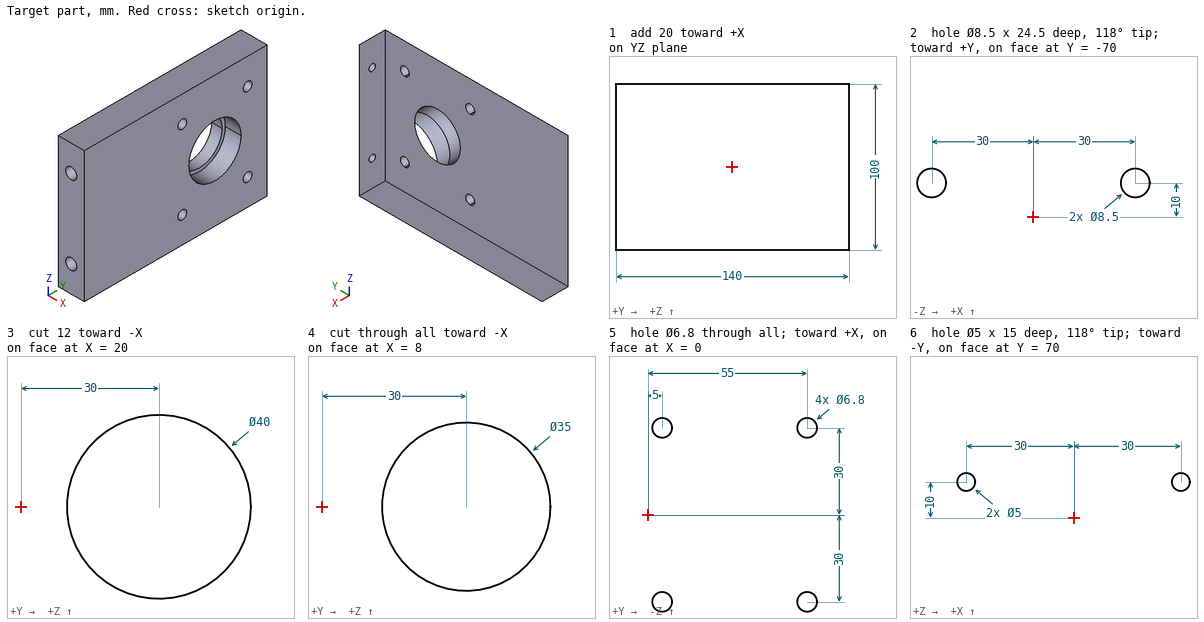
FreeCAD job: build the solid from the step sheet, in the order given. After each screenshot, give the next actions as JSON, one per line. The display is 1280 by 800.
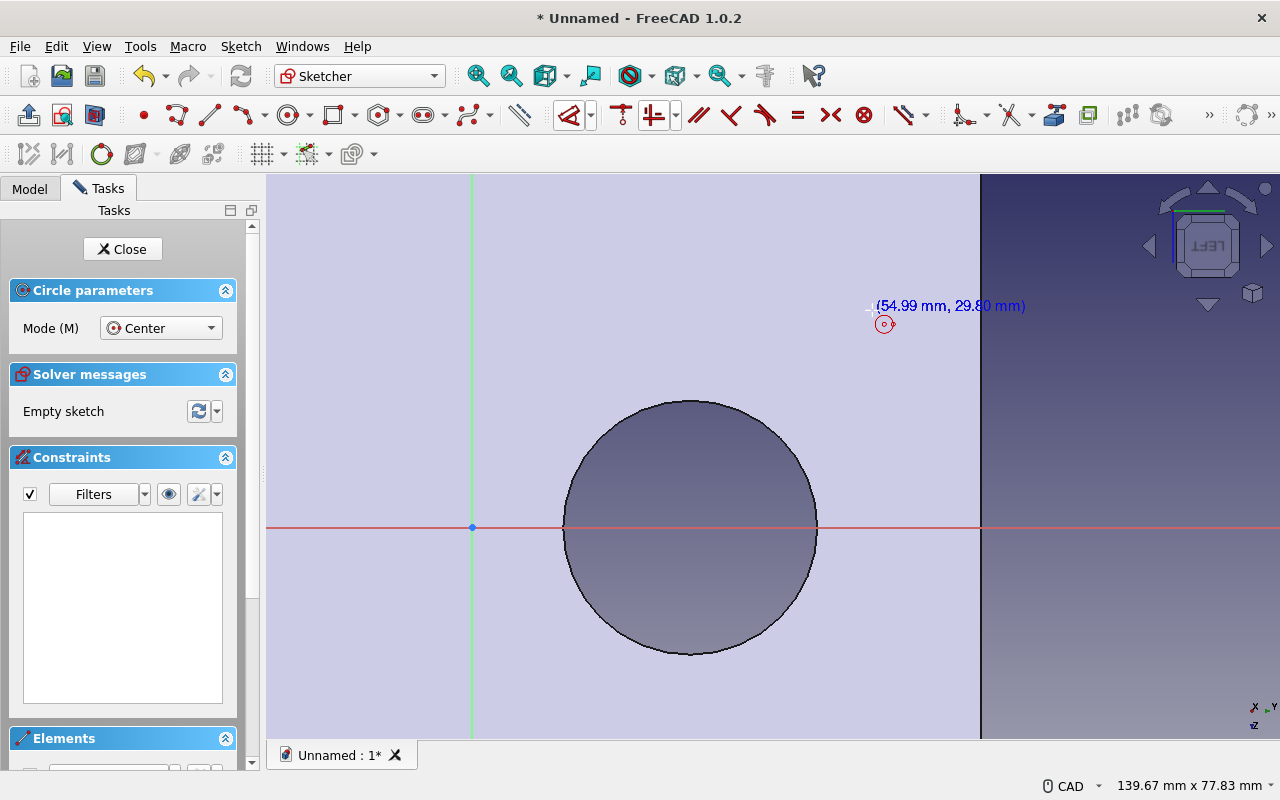
{"action": "left_click", "coordinate": [872, 310]}
{"action": "mouse_move", "coordinate": [889, 292]}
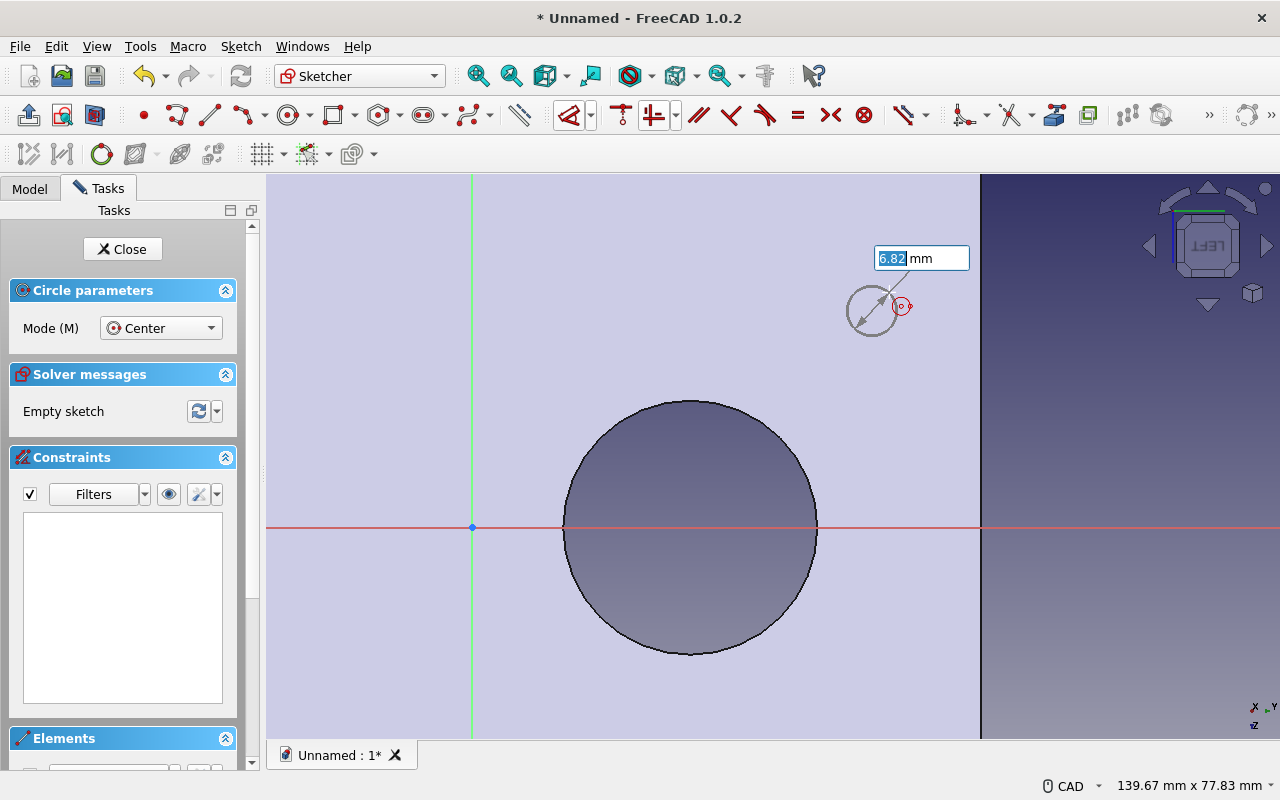
{"action": "type", "text": "6.8"}
{"action": "key", "text": "Return"}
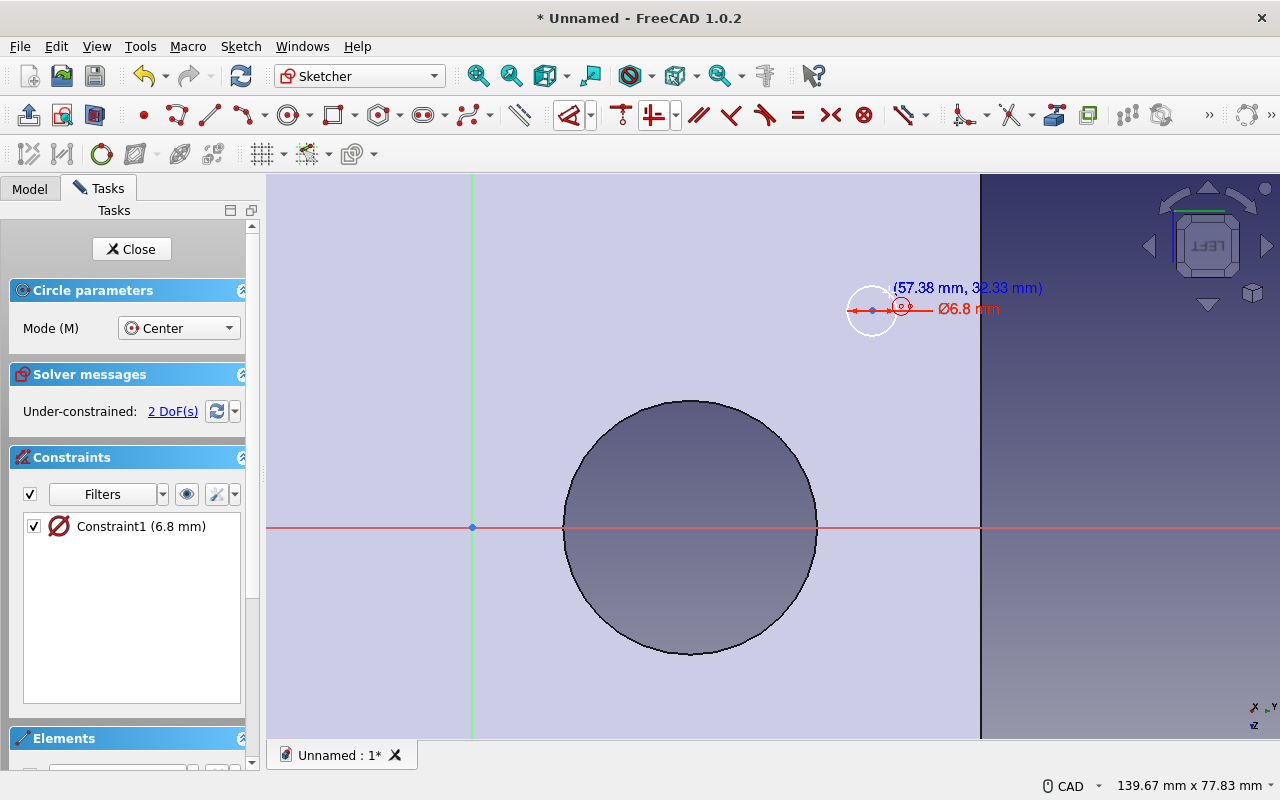
{"action": "scroll", "coordinate": [745, 312], "scroll_direction": "down", "scroll_amount": 2}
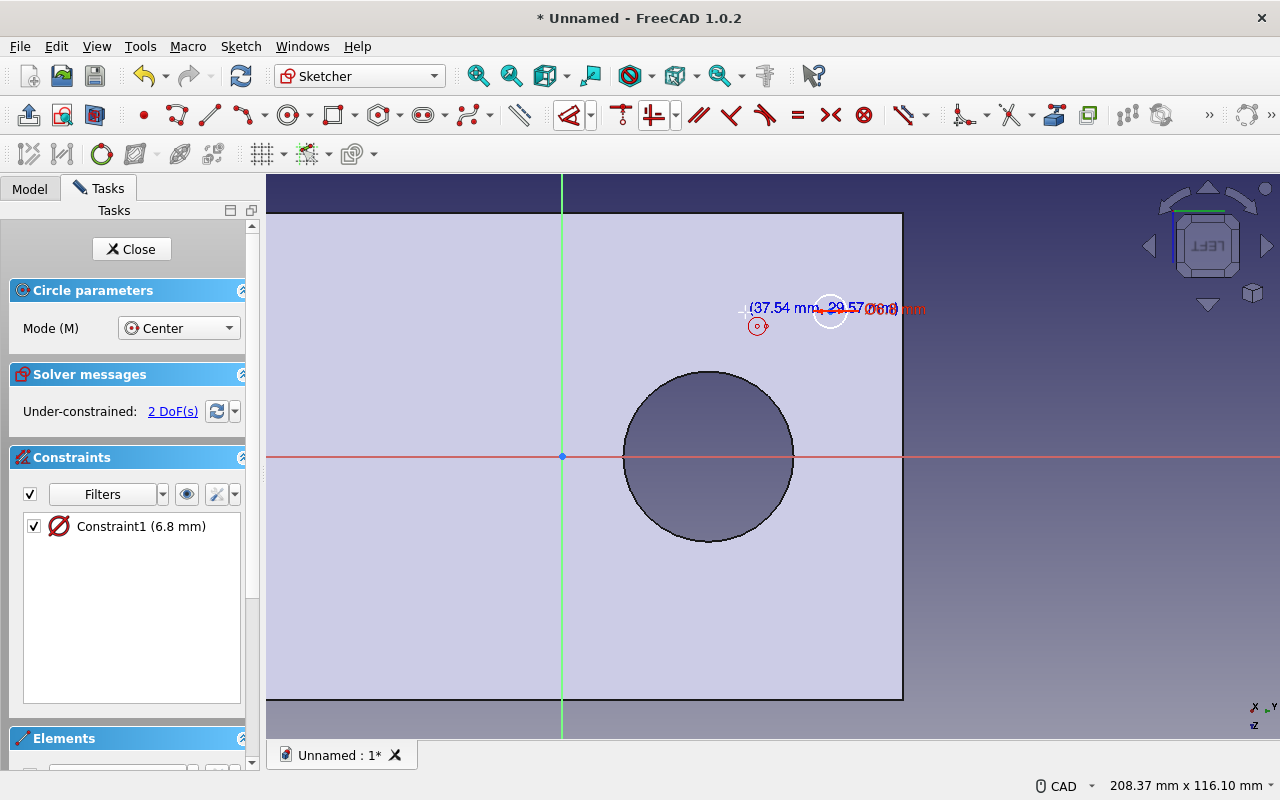
{"action": "scroll", "coordinate": [830, 603], "scroll_direction": "up", "scroll_amount": 2}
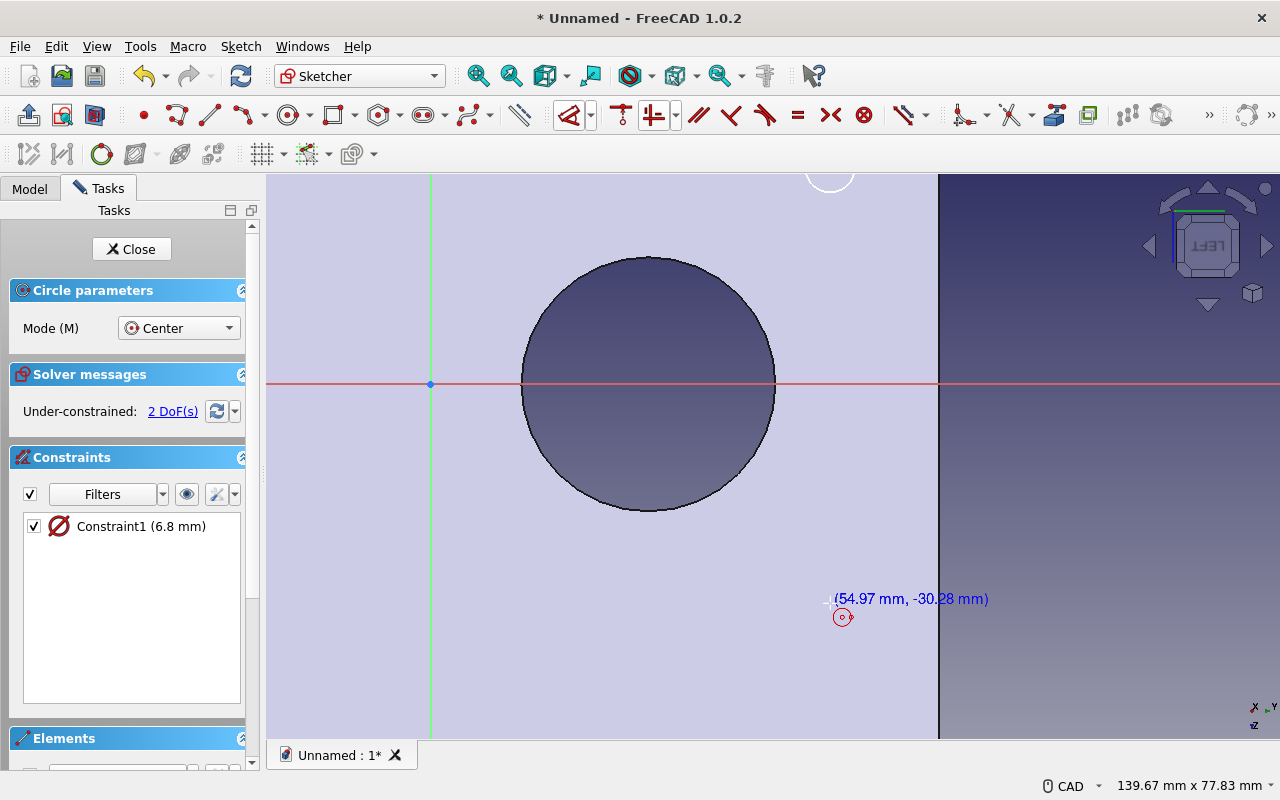
{"action": "left_click", "coordinate": [830, 602]}
{"action": "mouse_move", "coordinate": [847, 585]}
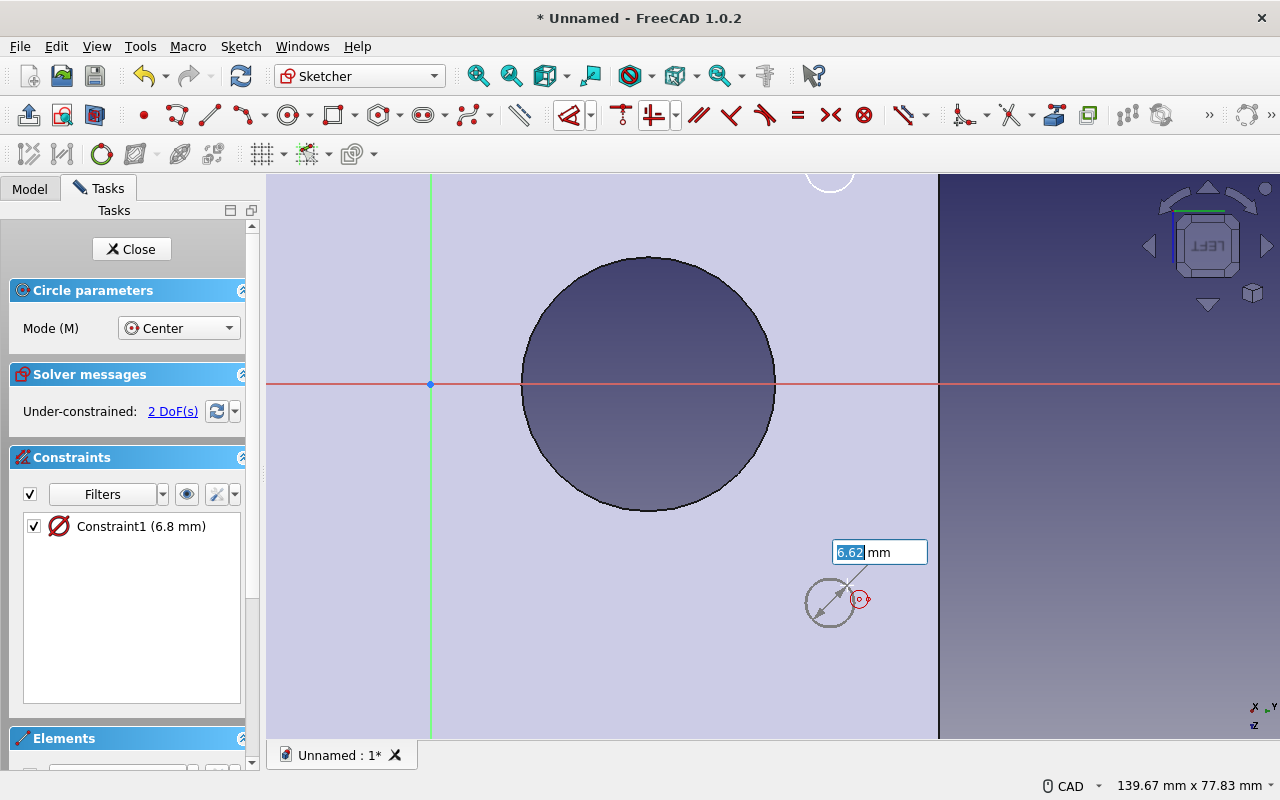
{"action": "type", "text": "6.8"}
{"action": "key", "text": "Return"}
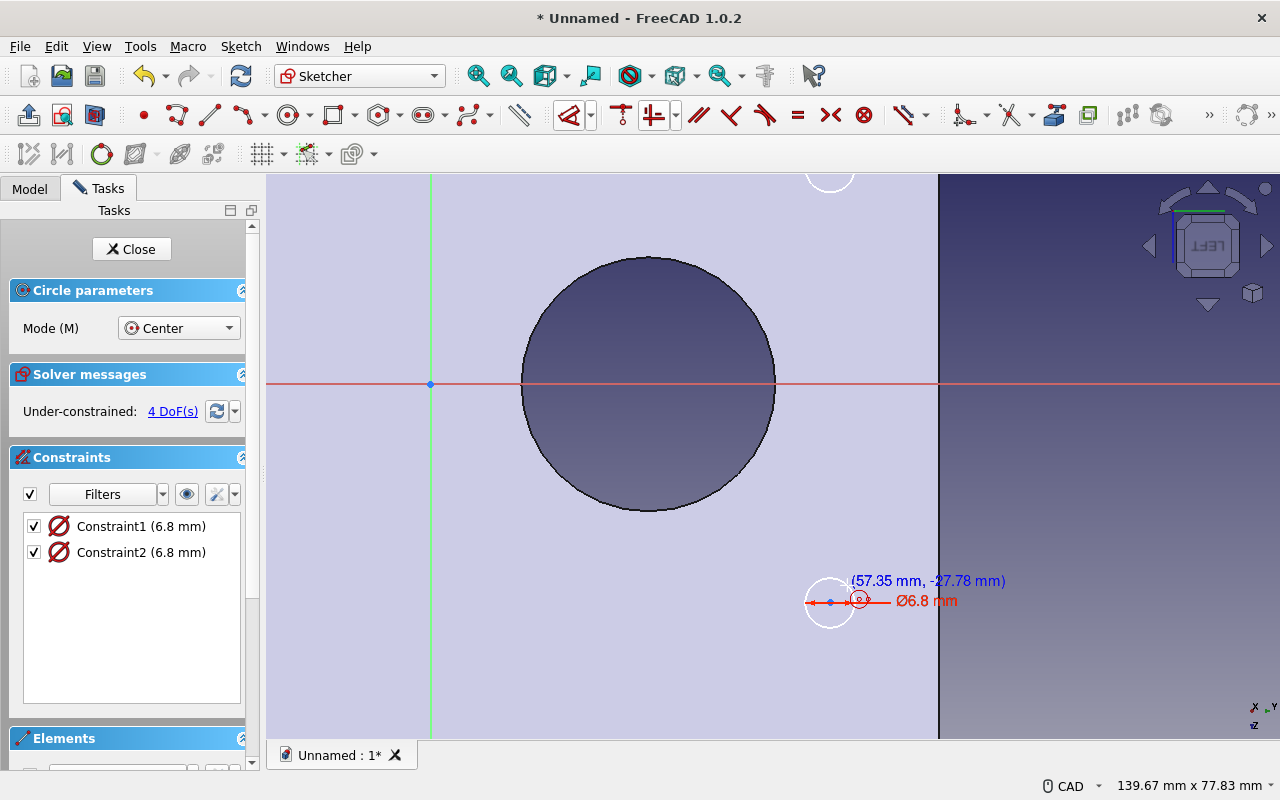
{"action": "scroll", "coordinate": [830, 603], "scroll_direction": "down", "scroll_amount": 2}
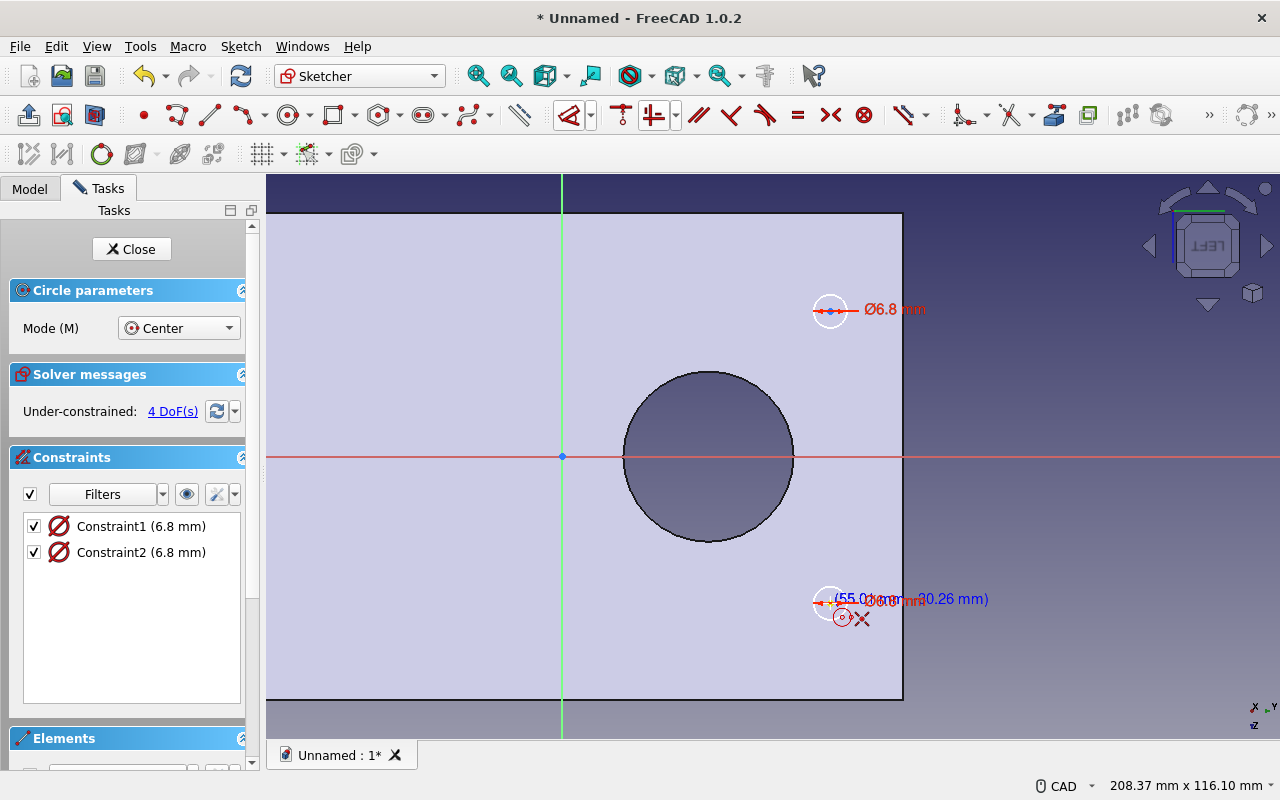
{"action": "scroll", "coordinate": [587, 311], "scroll_direction": "up", "scroll_amount": 2}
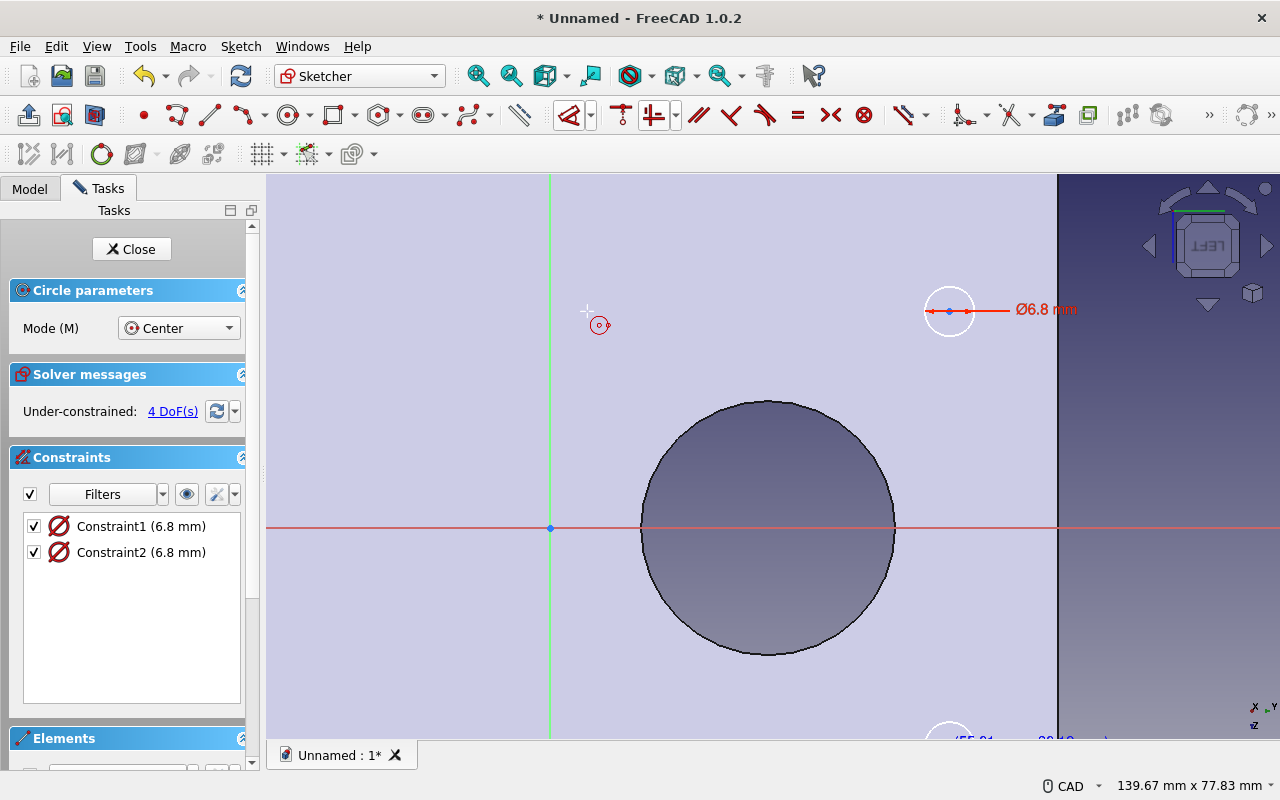
{"action": "left_click", "coordinate": [587, 310]}
{"action": "mouse_move", "coordinate": [604, 293]}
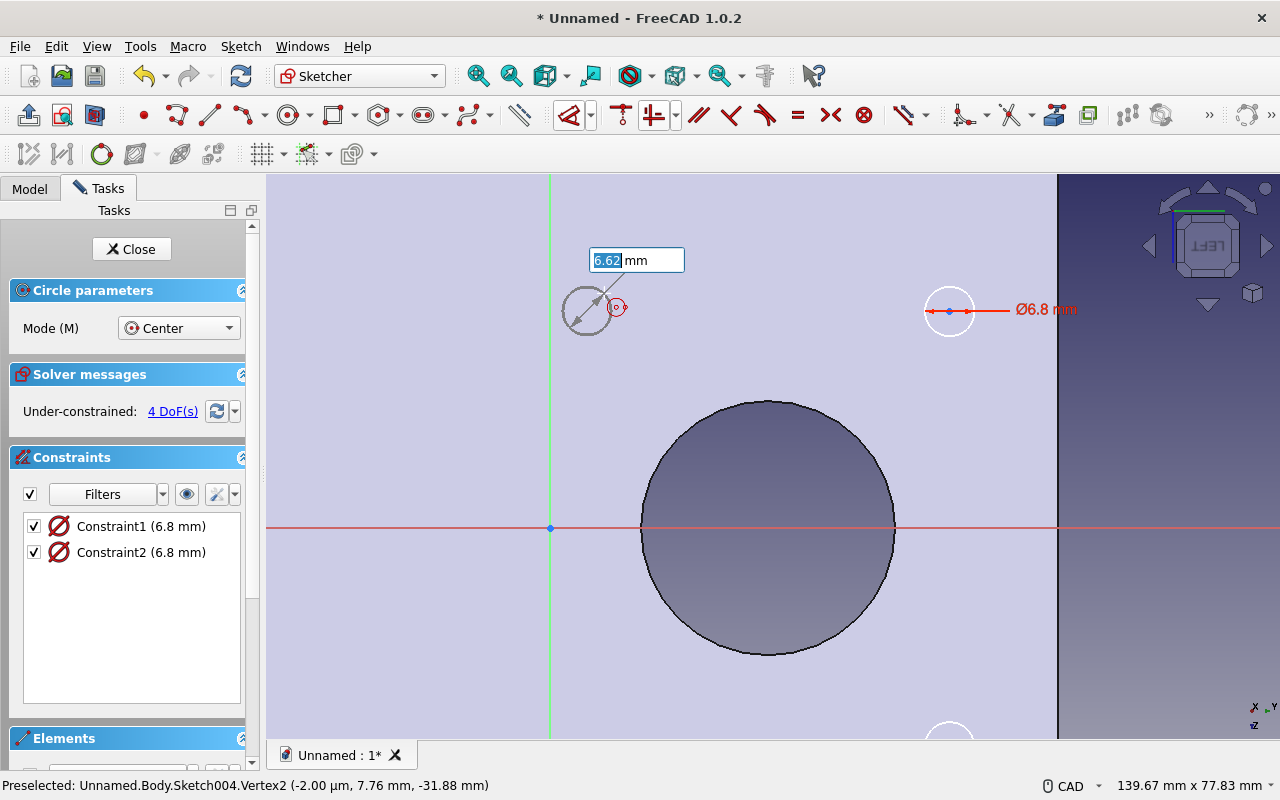
{"action": "type", "text": "6.8"}
{"action": "key", "text": "Return"}